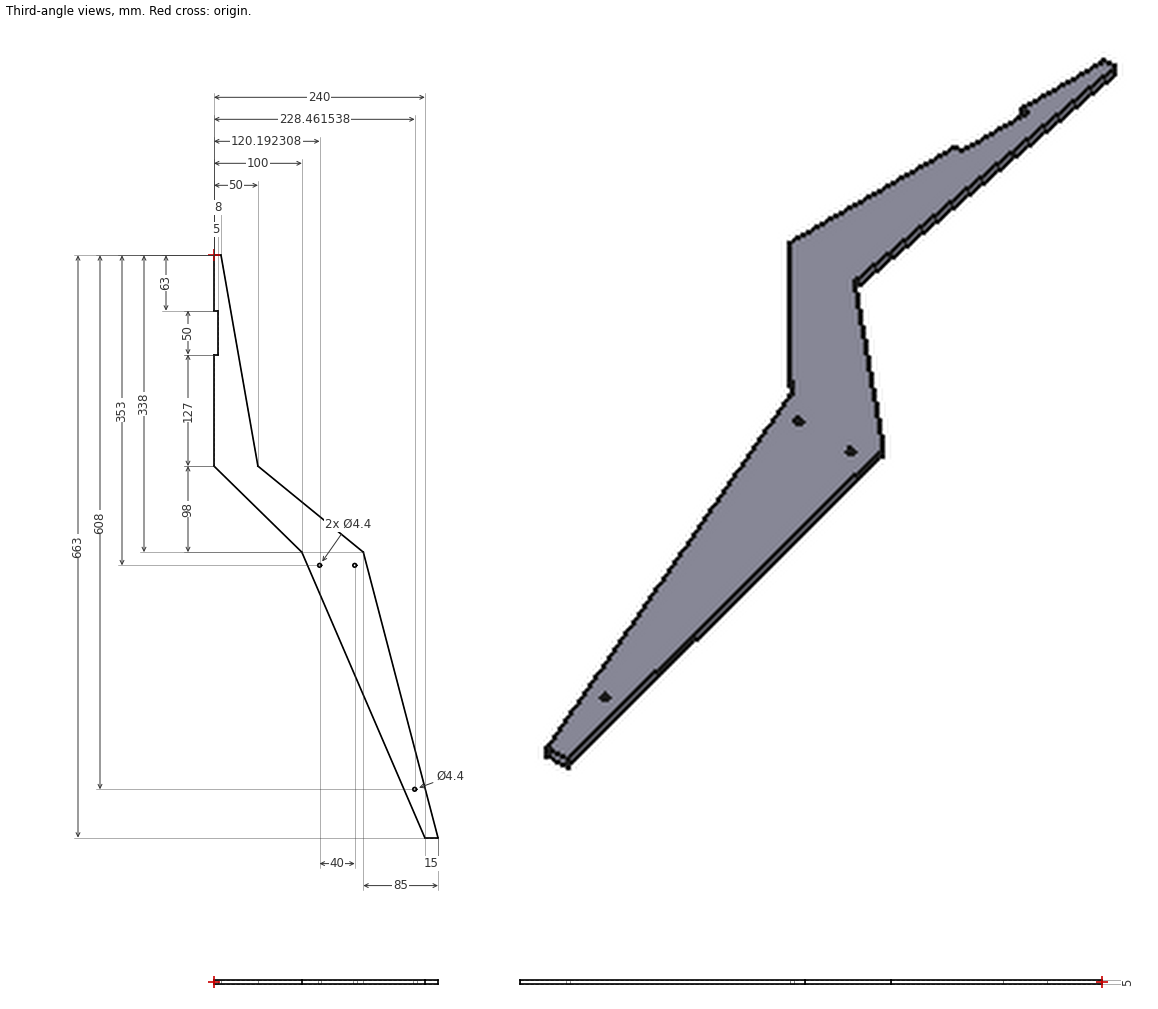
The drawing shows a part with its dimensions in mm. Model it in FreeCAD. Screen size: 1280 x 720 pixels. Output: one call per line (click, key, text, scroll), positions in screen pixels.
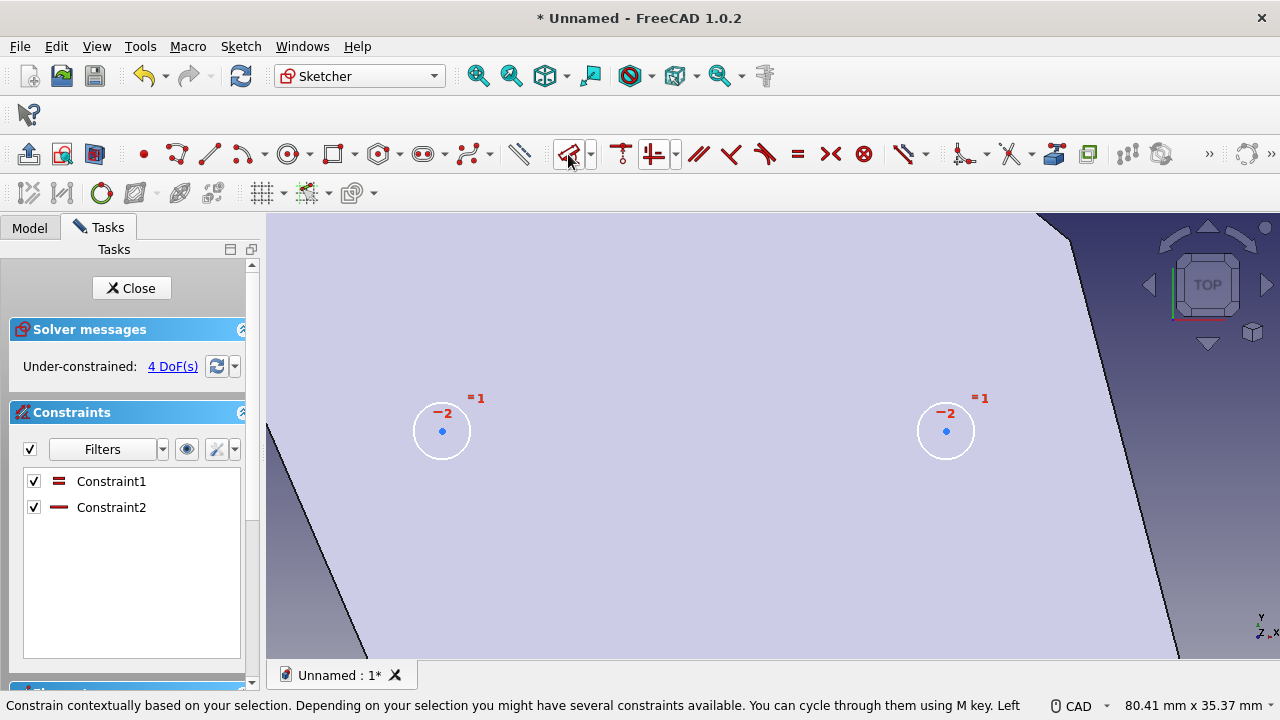
click(462, 411)
click(485, 388)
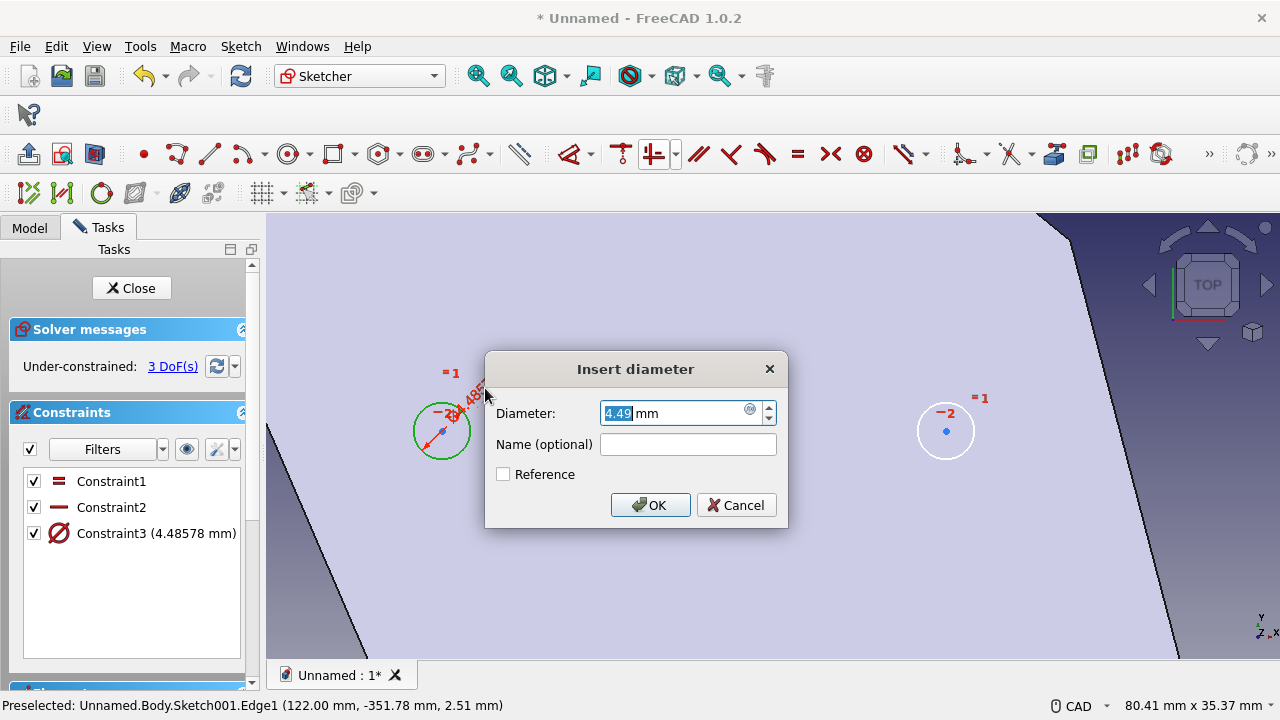
text(4.4)
key(Return)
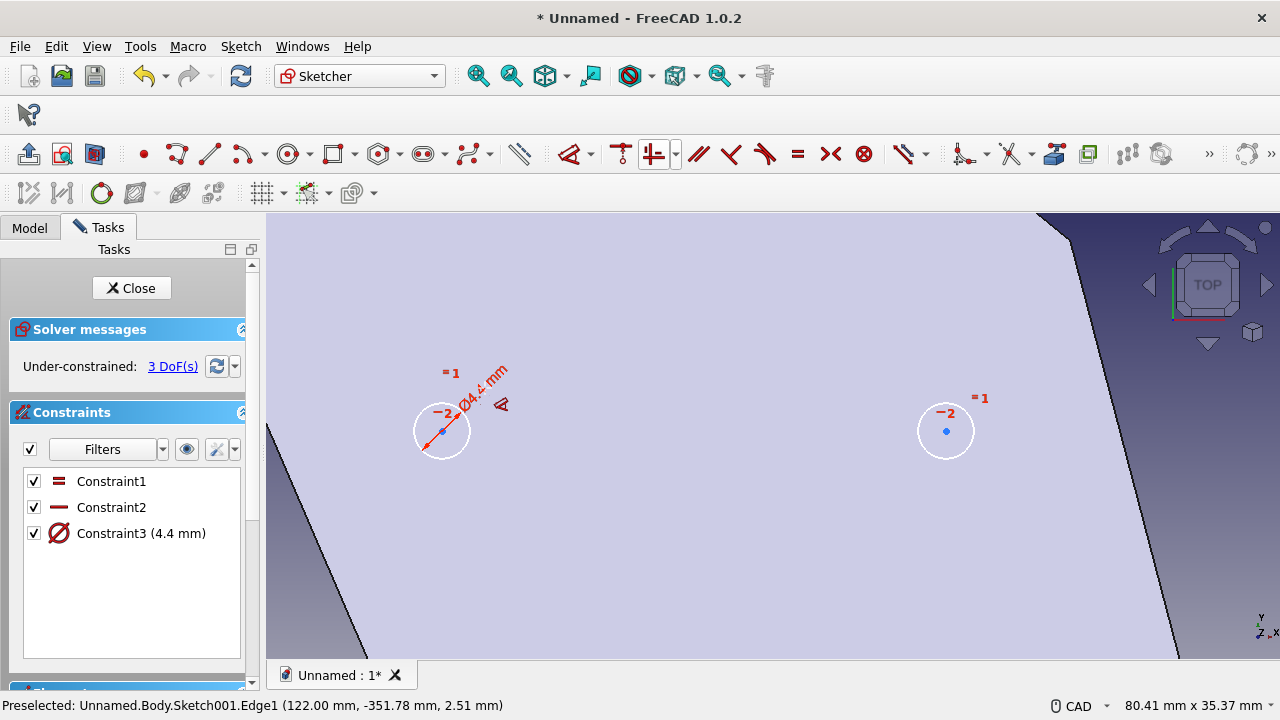
click(442, 431)
click(476, 336)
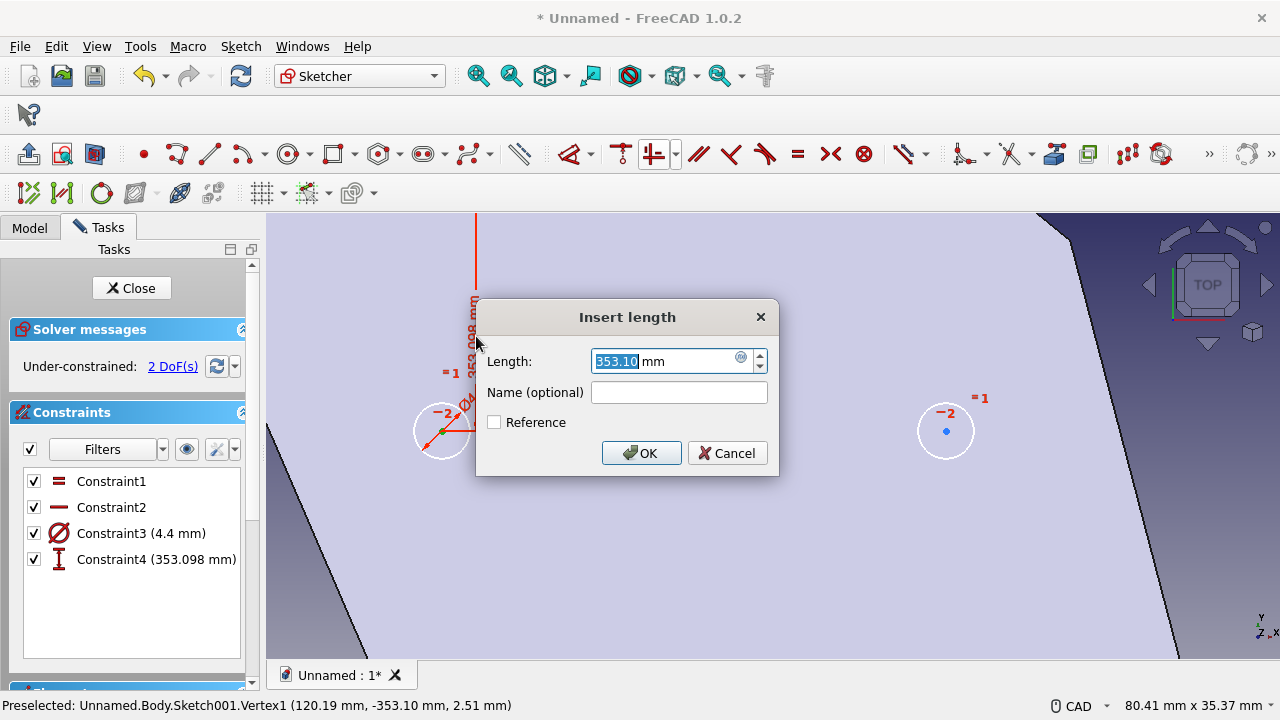
text(353)
key(Return)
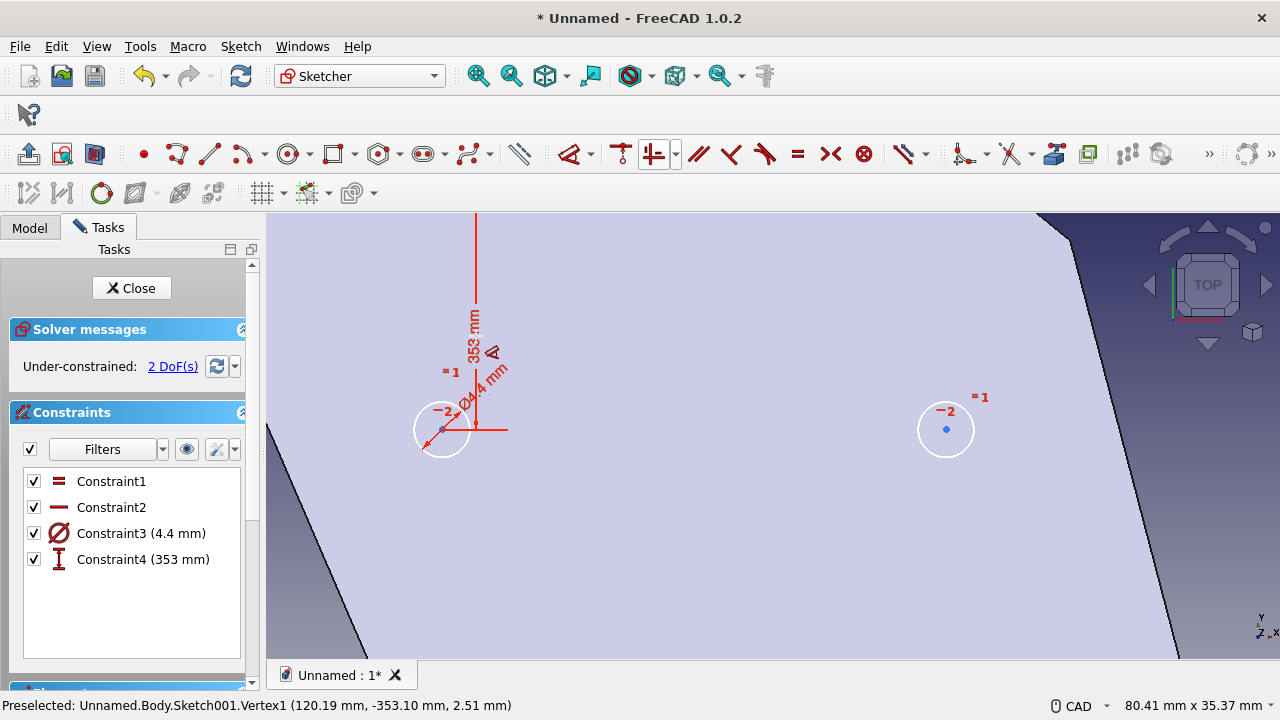
click(442, 430)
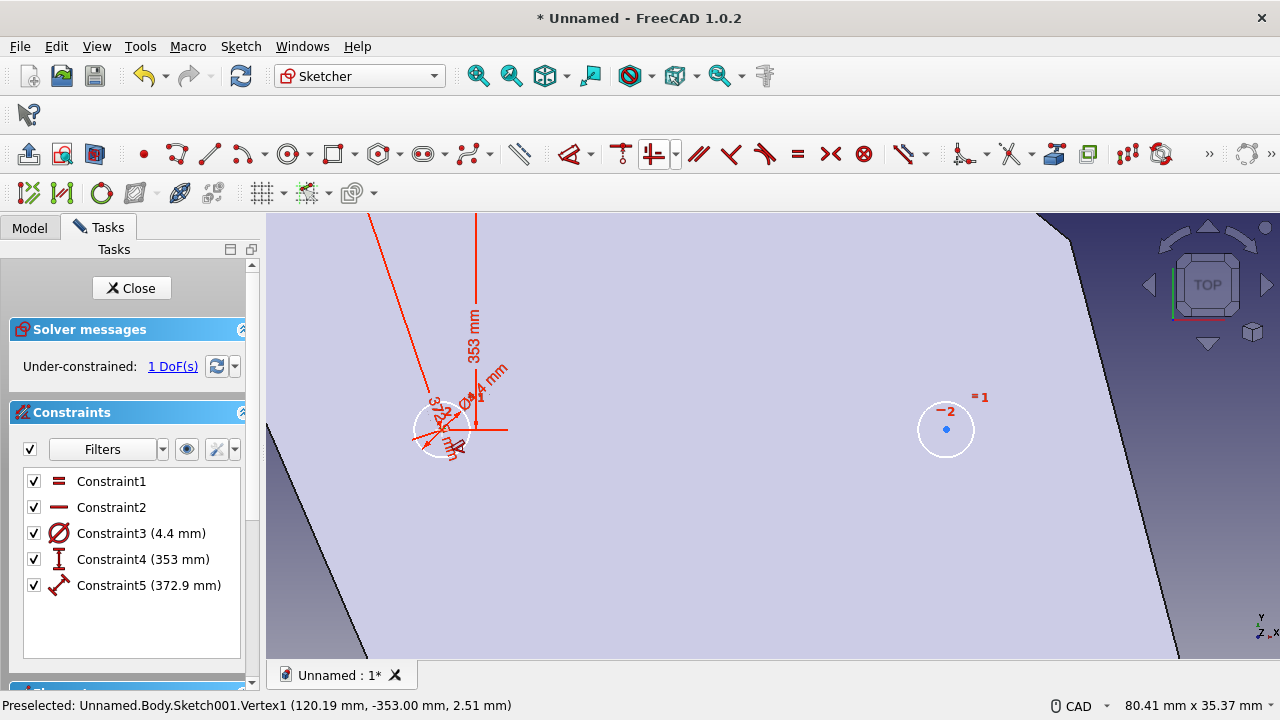
click(946, 430)
click(694, 464)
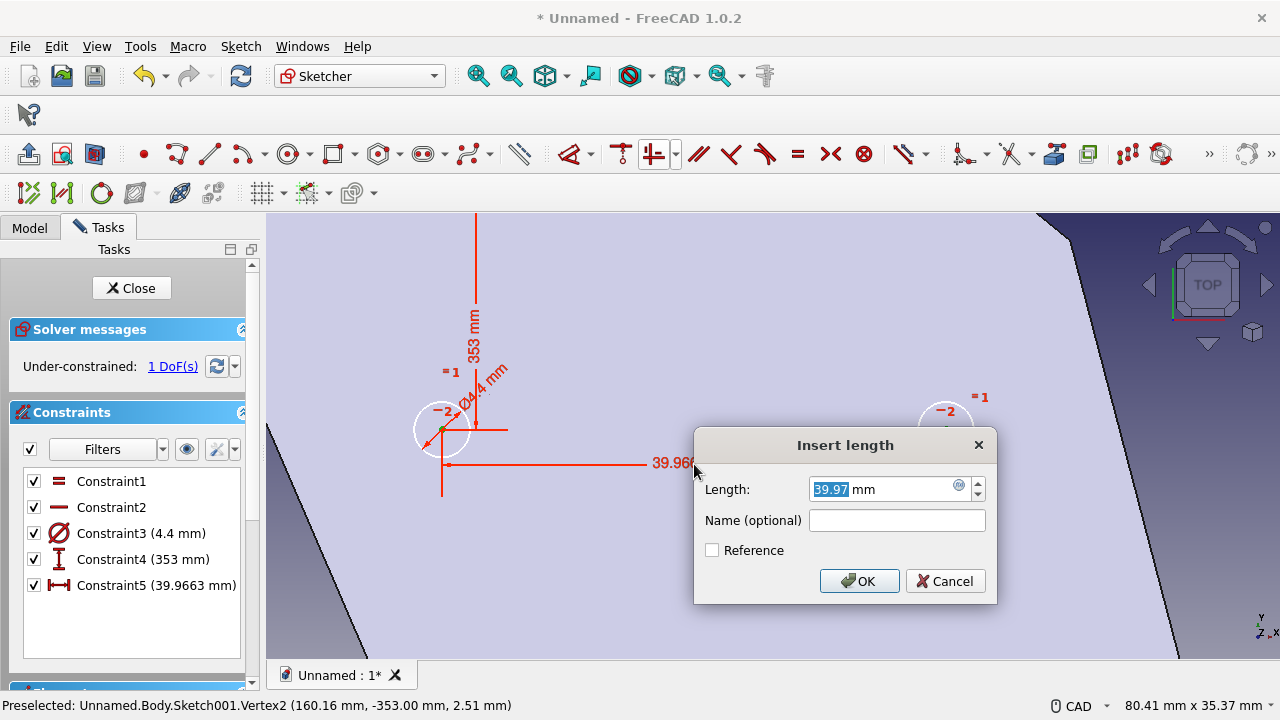
text(40)
key(Return)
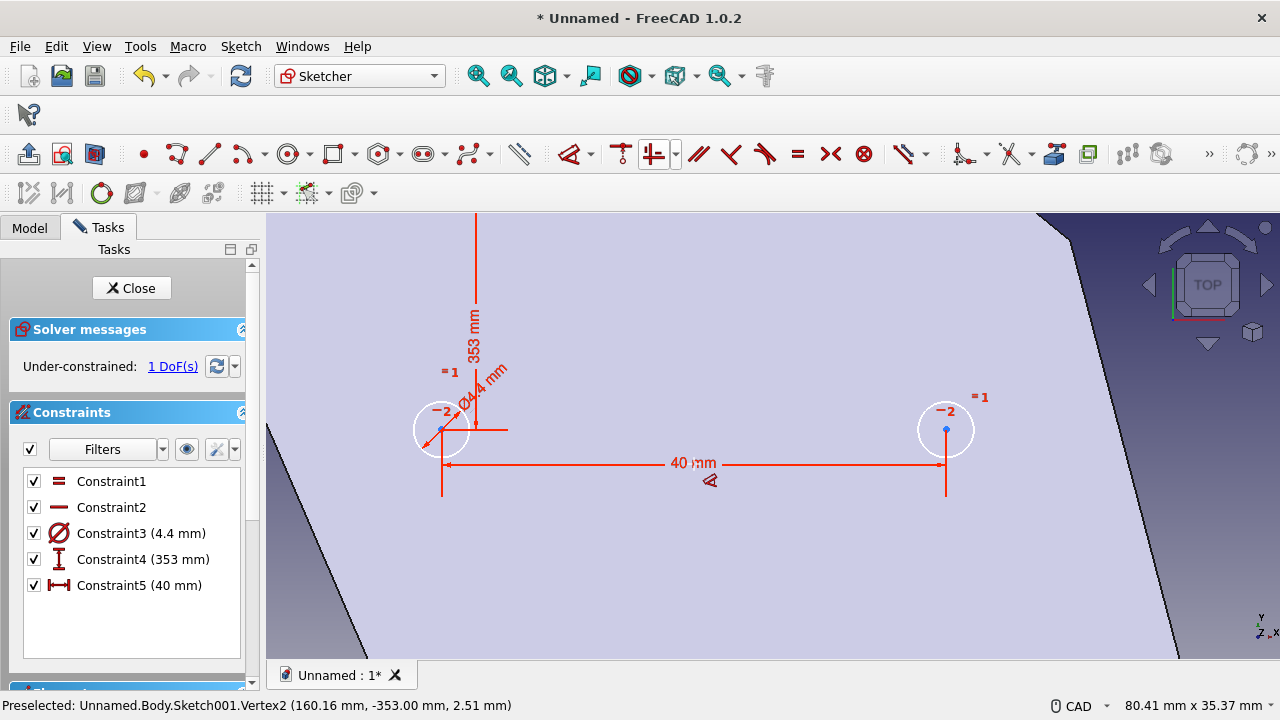
click(442, 430)
click(368, 464)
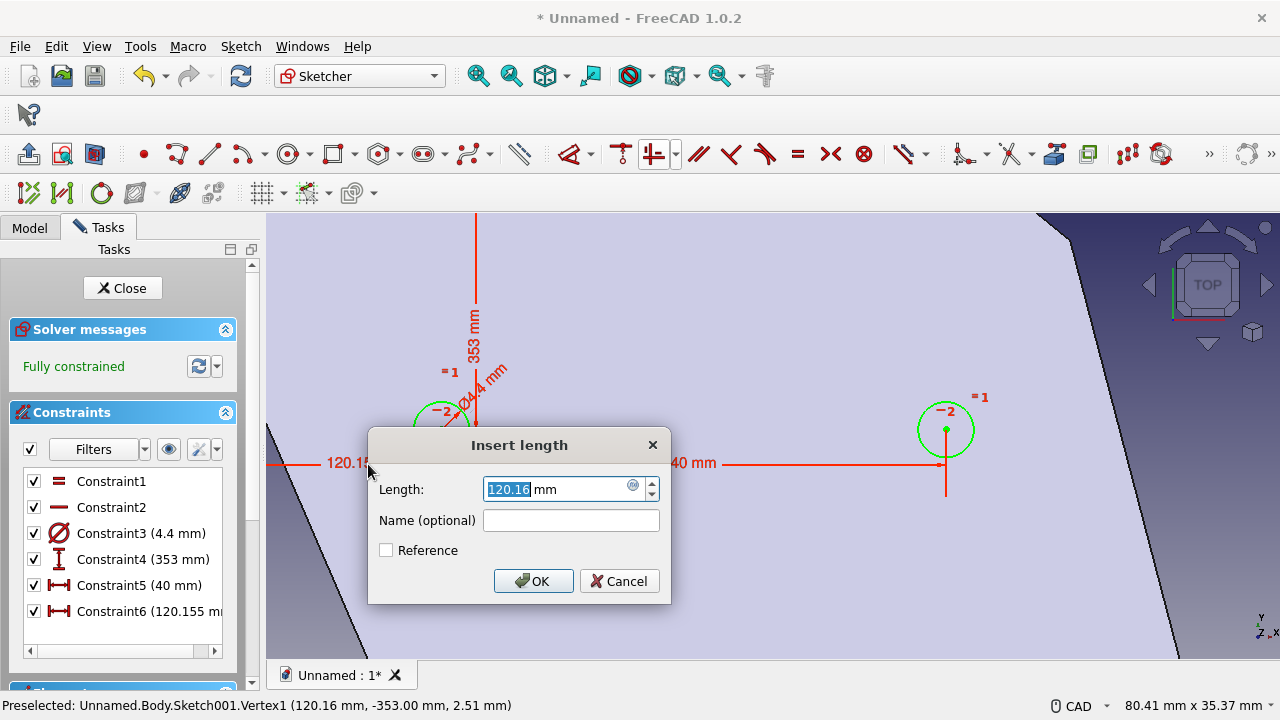
text(120.192308)
key(Return)
key(Escape)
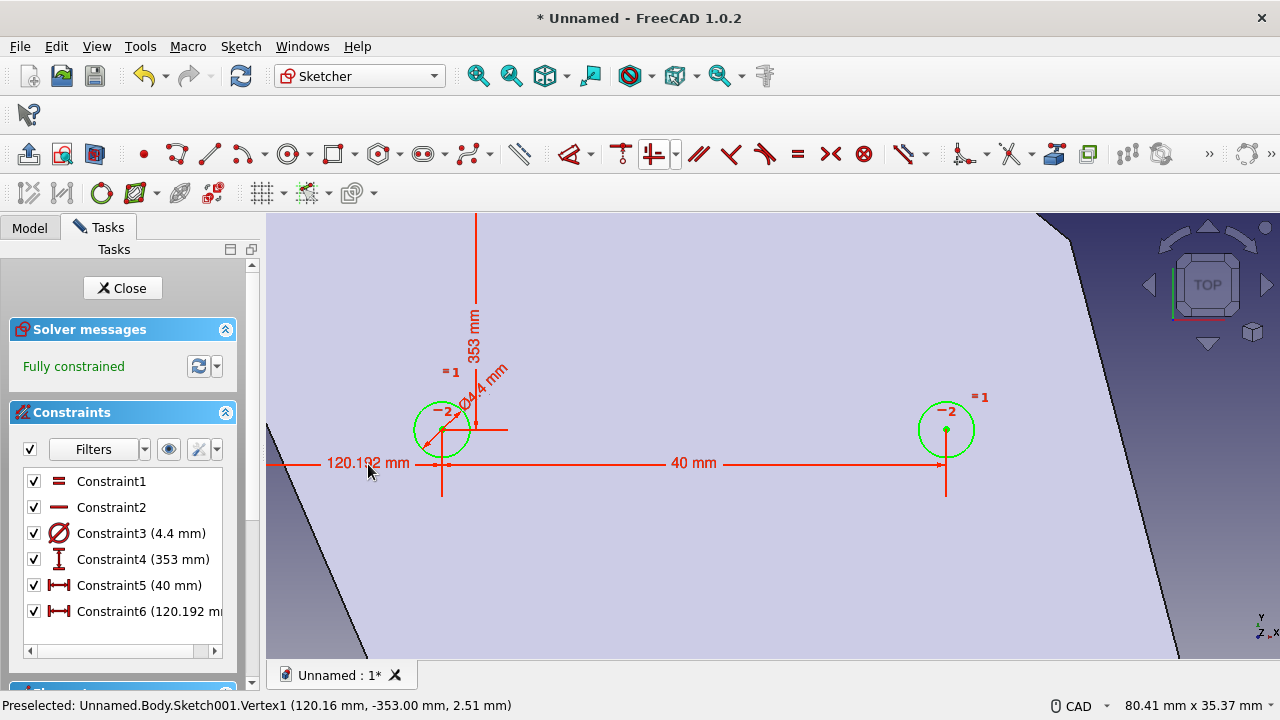
click(123, 288)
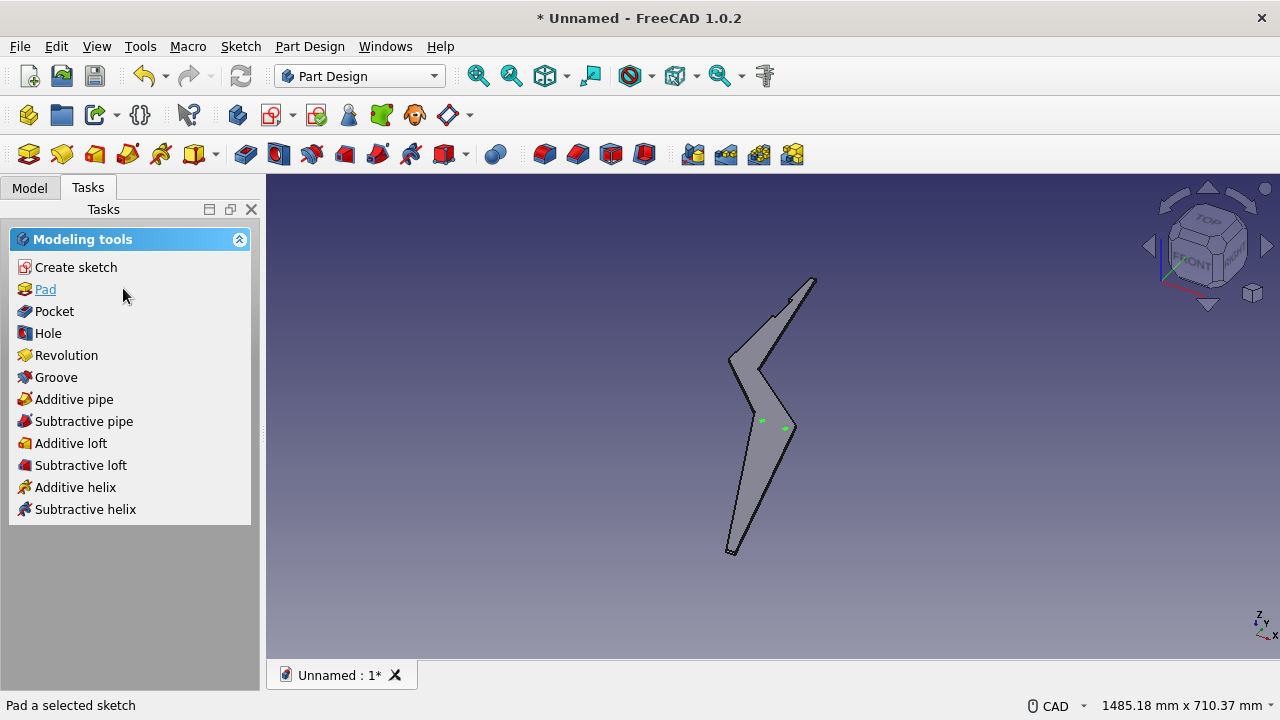
click(246, 154)